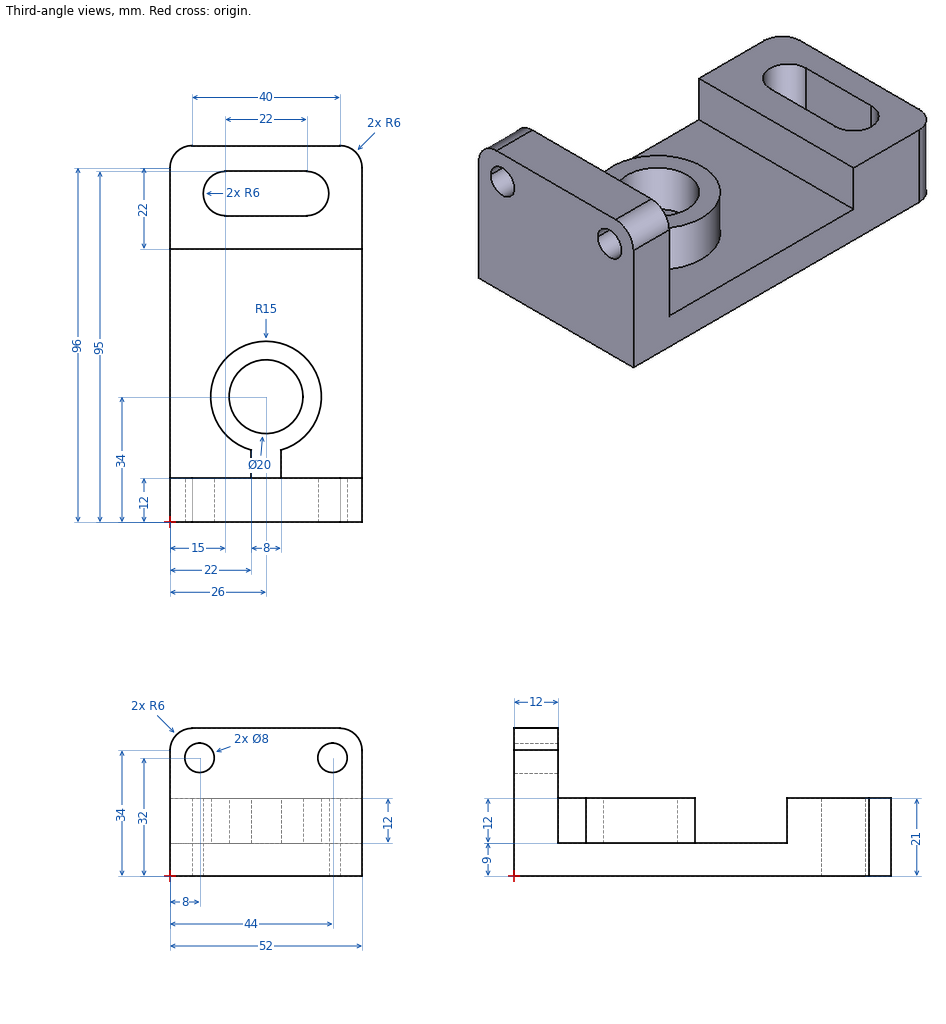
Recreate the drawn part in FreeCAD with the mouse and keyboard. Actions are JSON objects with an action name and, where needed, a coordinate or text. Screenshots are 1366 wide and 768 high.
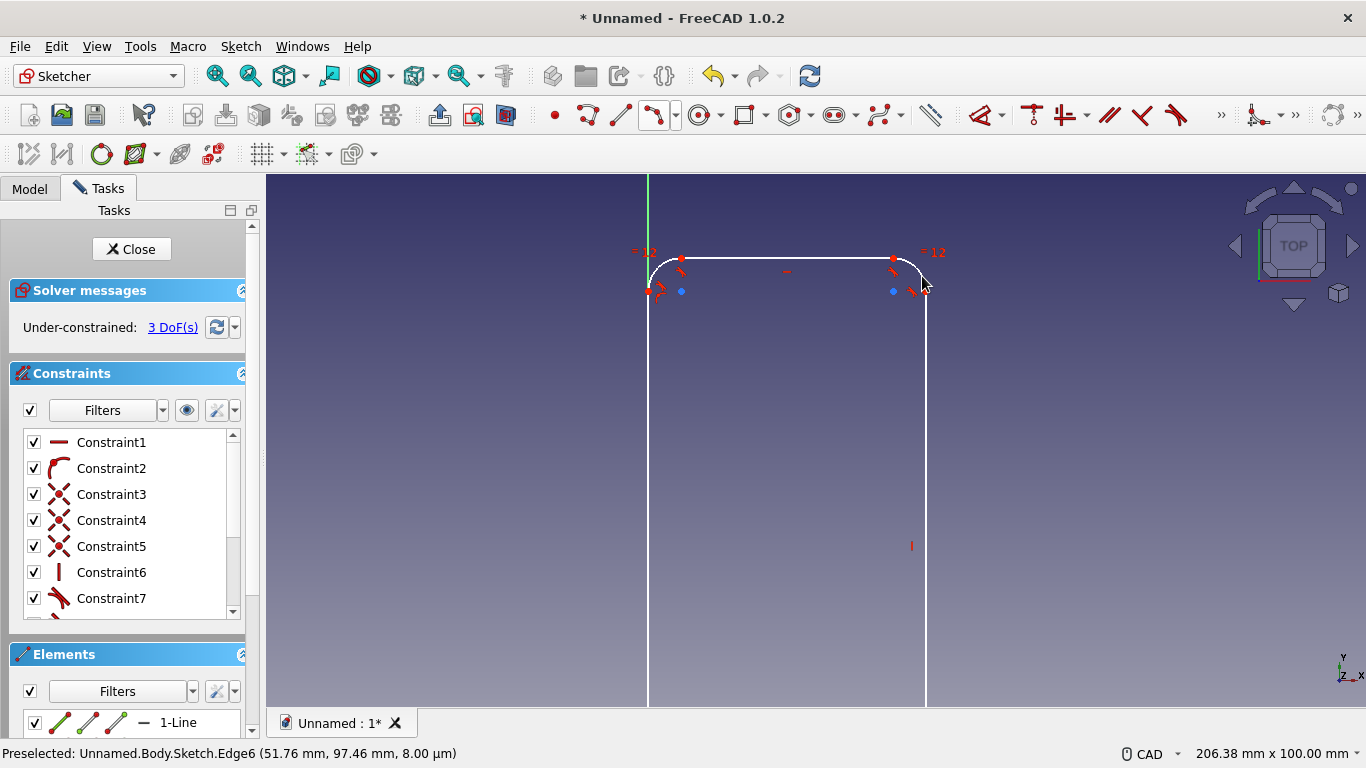
{"action": "scroll", "coordinate": [666, 262], "scroll_direction": "up", "scroll_amount": 2}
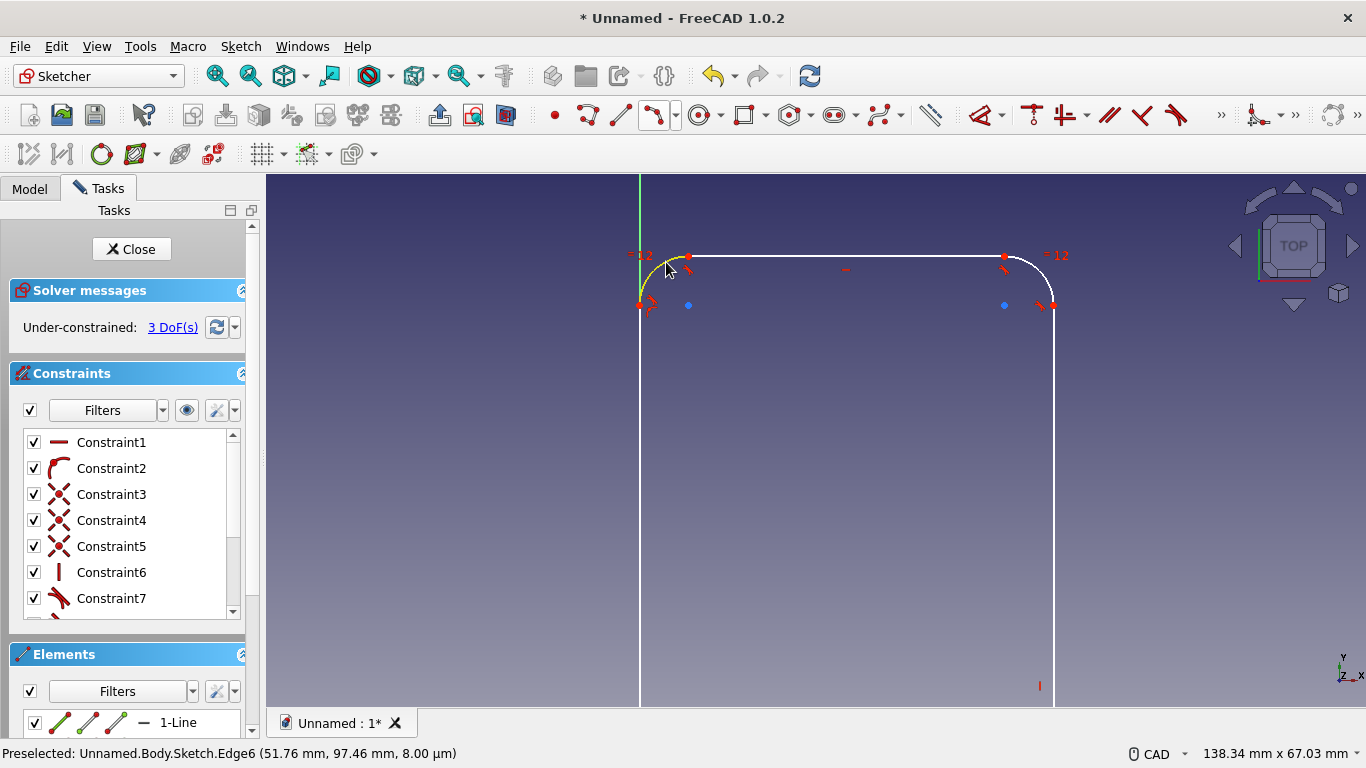
{"action": "left_click", "coordinate": [666, 262]}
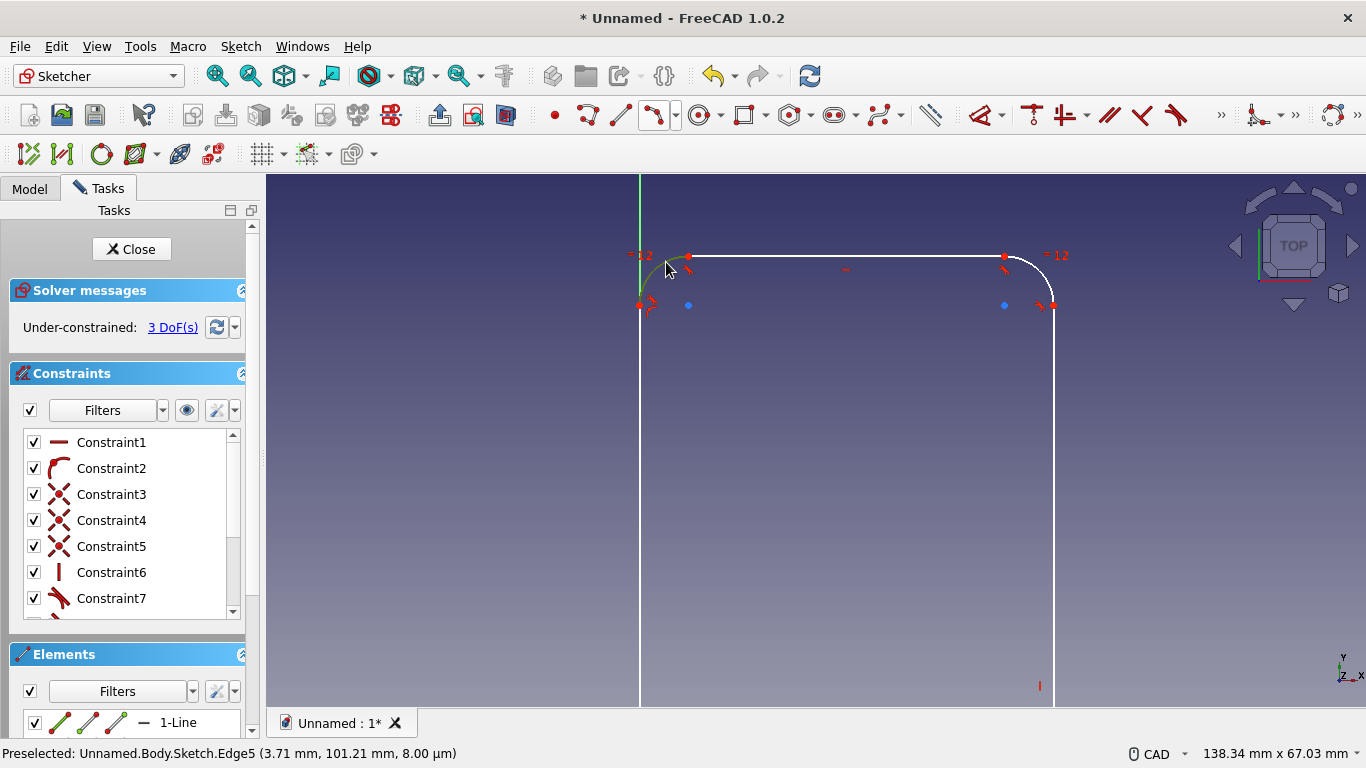
{"action": "key", "text": "k r"}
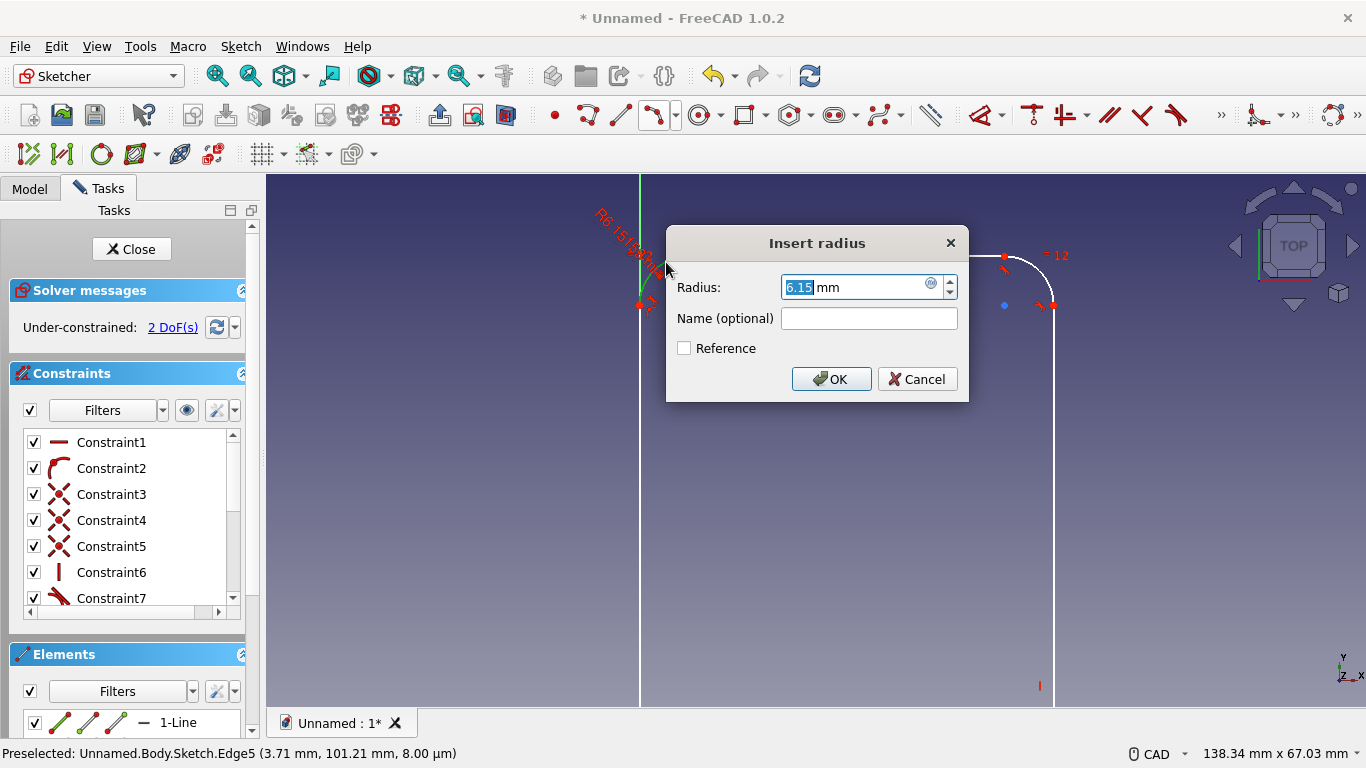
{"action": "type", "text": "6"}
{"action": "key", "text": "Return"}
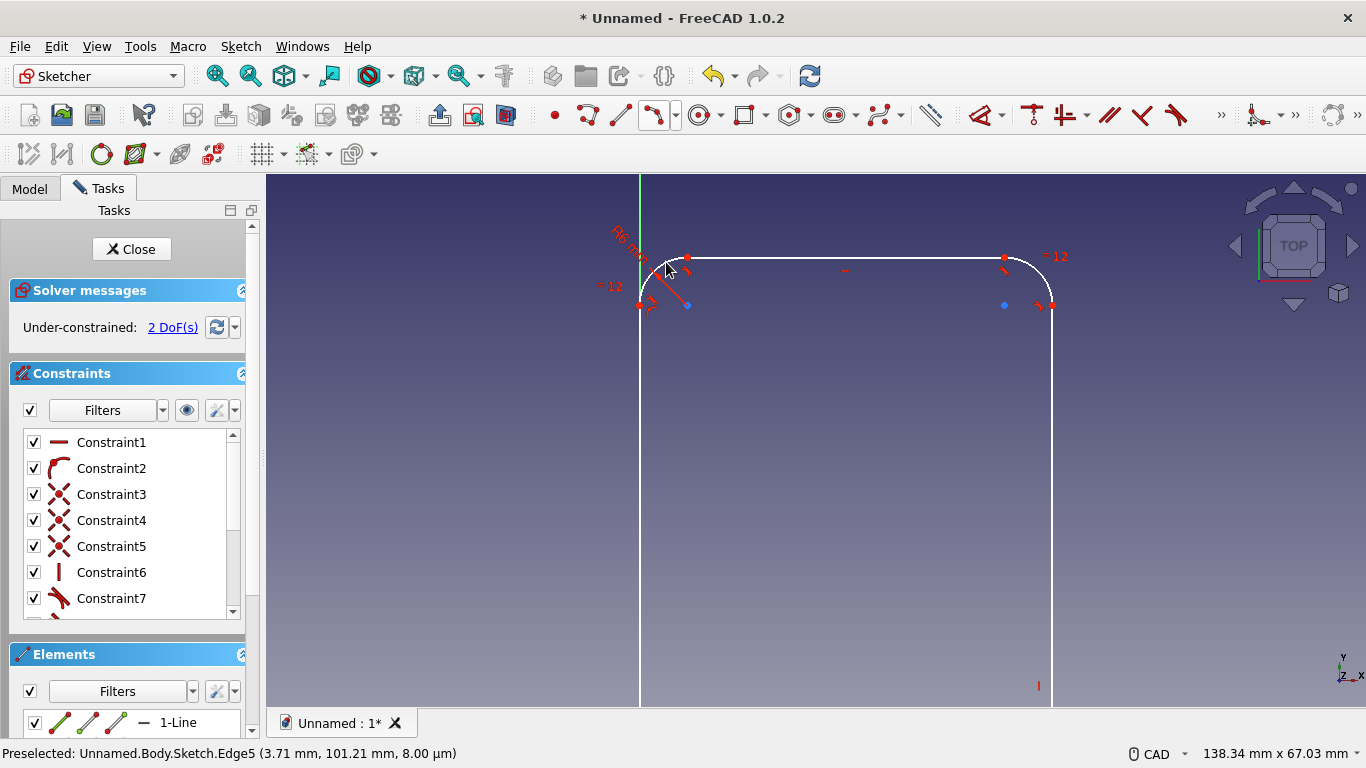
{"action": "left_click", "coordinate": [909, 258]}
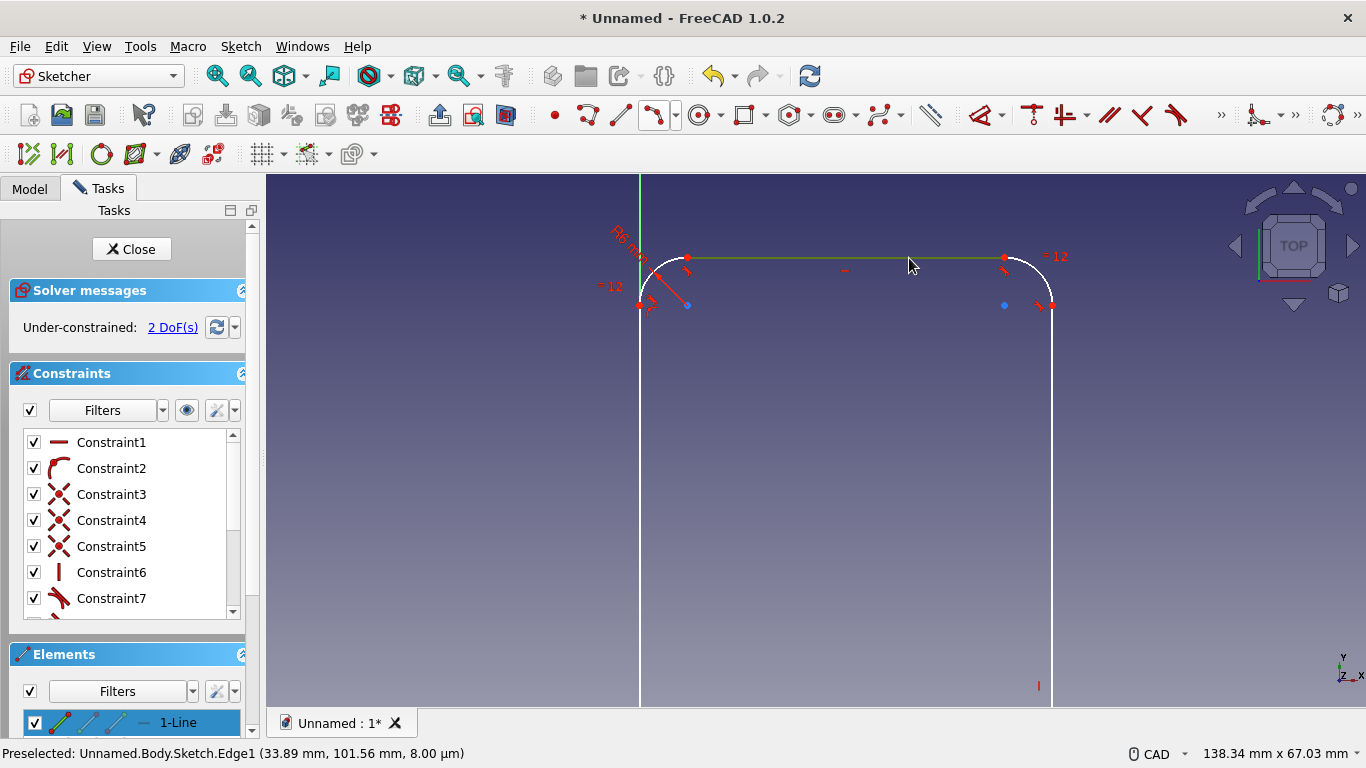
{"action": "left_click", "coordinate": [1002, 116]}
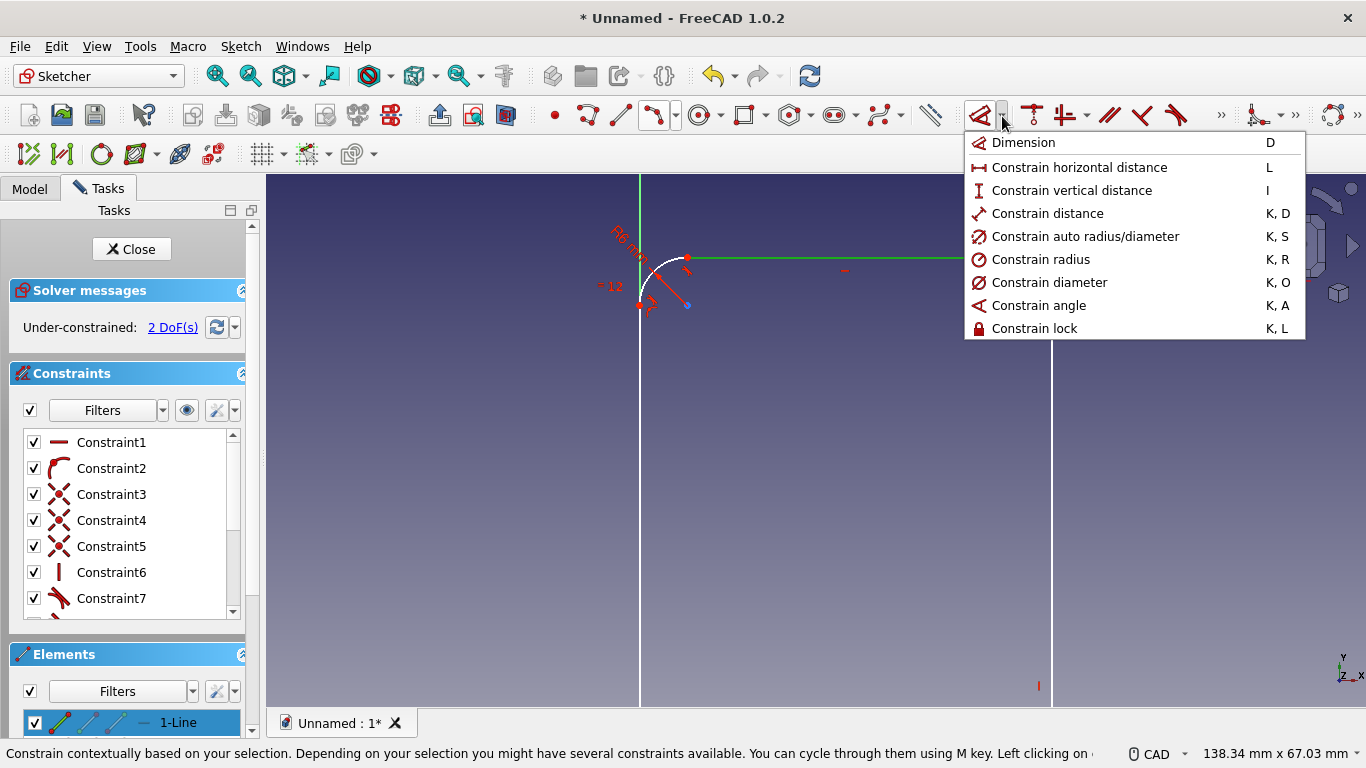
{"action": "left_click", "coordinate": [1135, 168]}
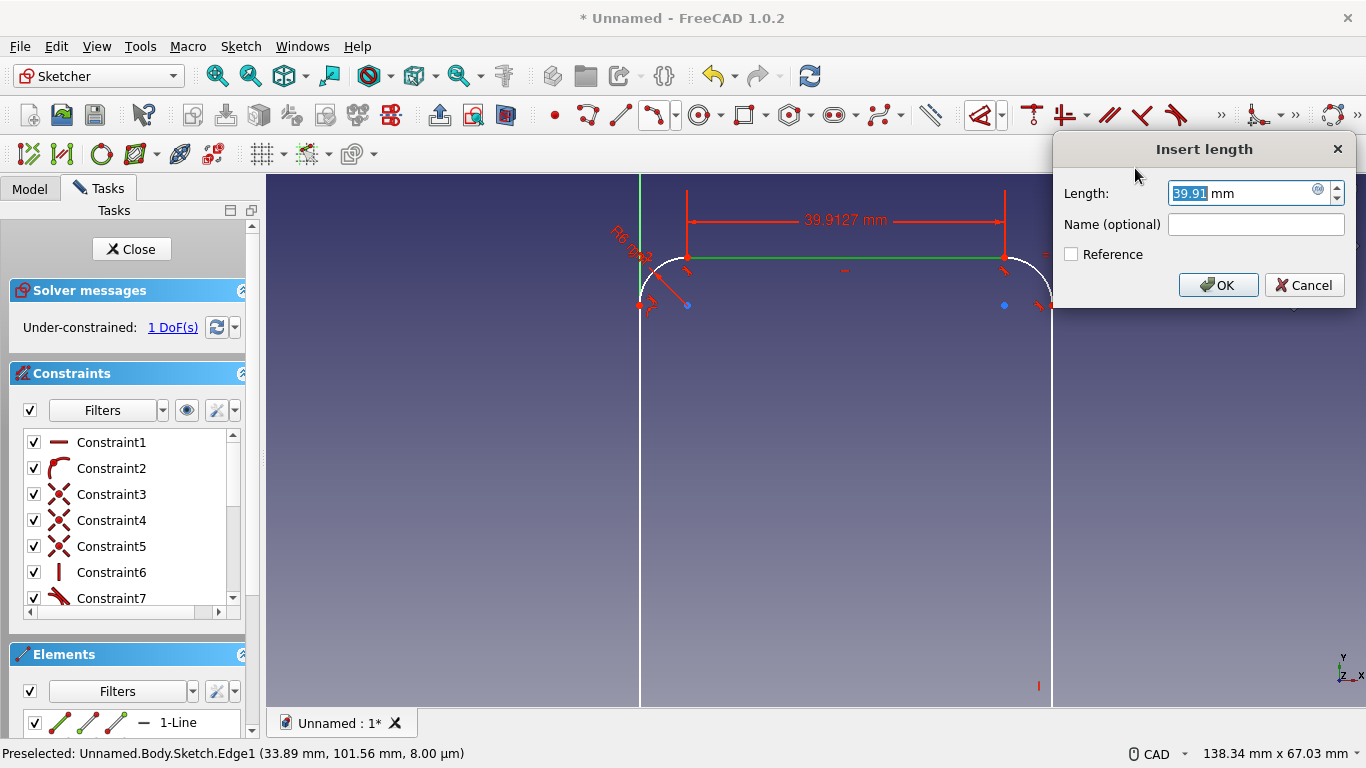
{"action": "type", "text": "40"}
{"action": "key", "text": "Return"}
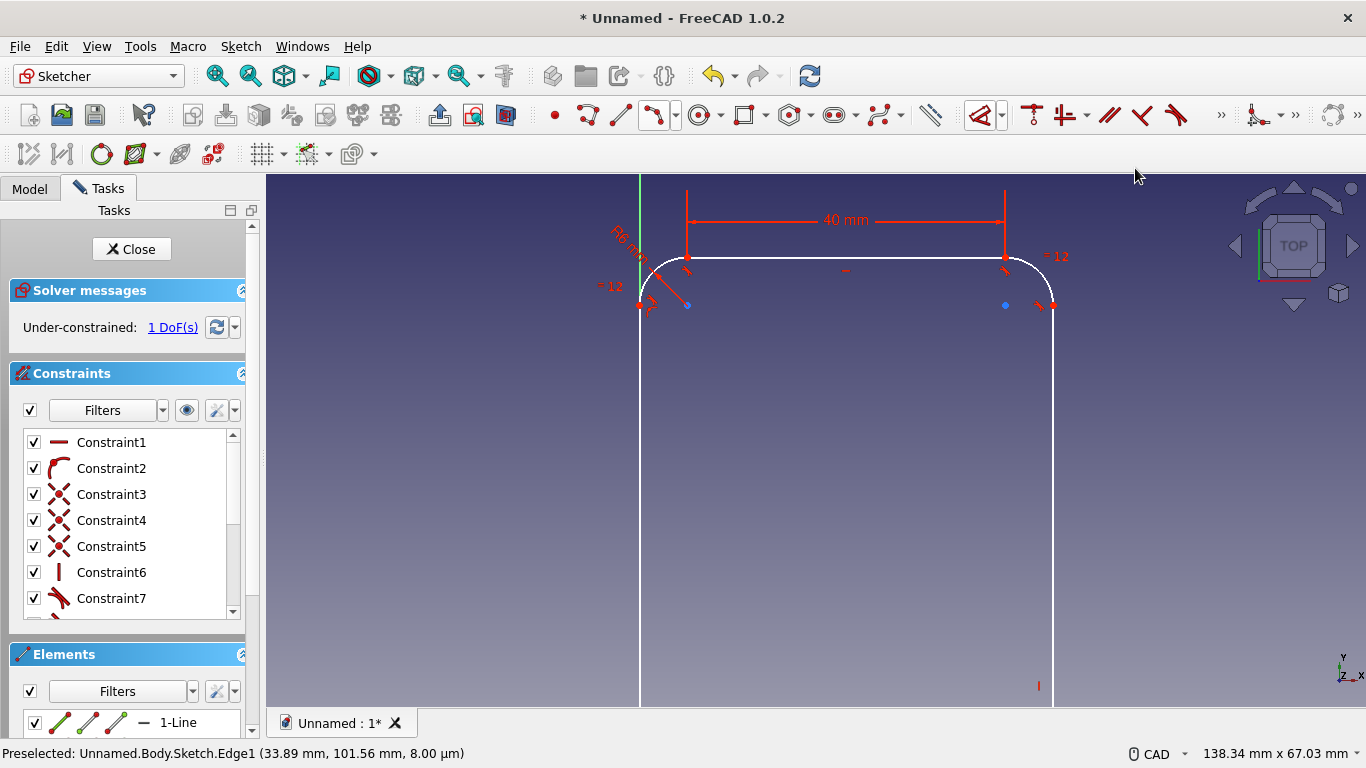
{"action": "left_click", "coordinate": [640, 533]}